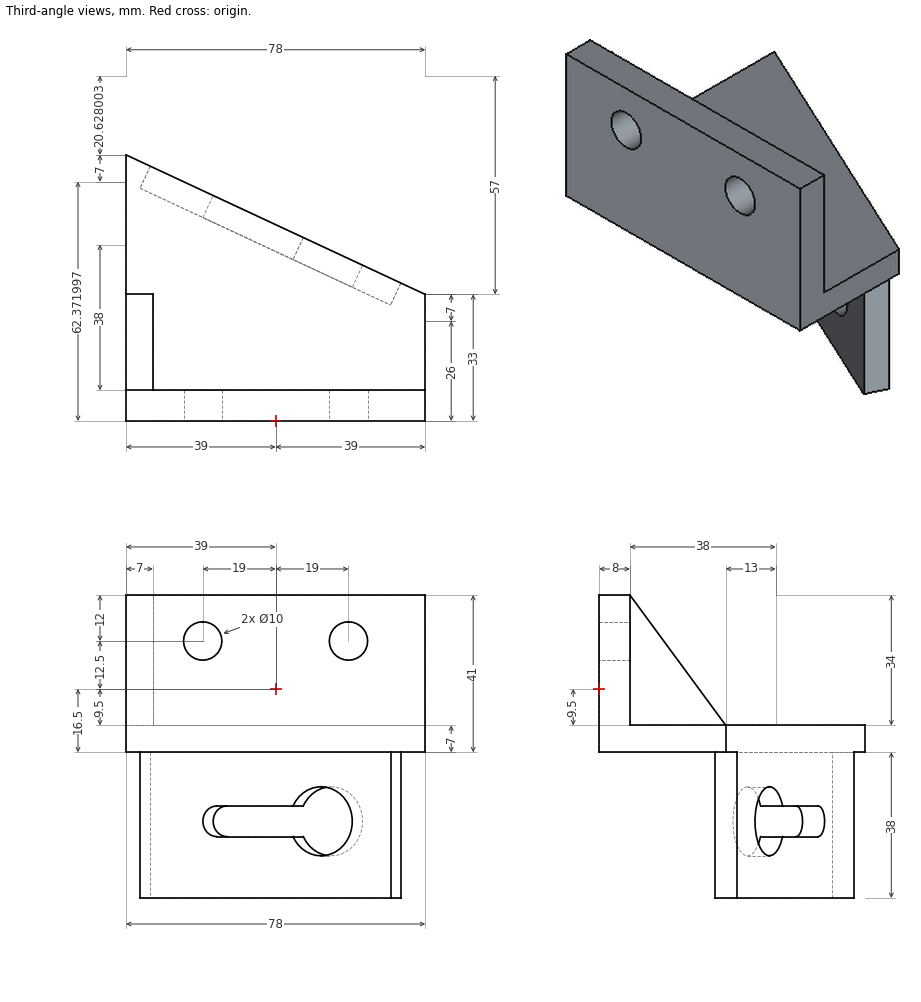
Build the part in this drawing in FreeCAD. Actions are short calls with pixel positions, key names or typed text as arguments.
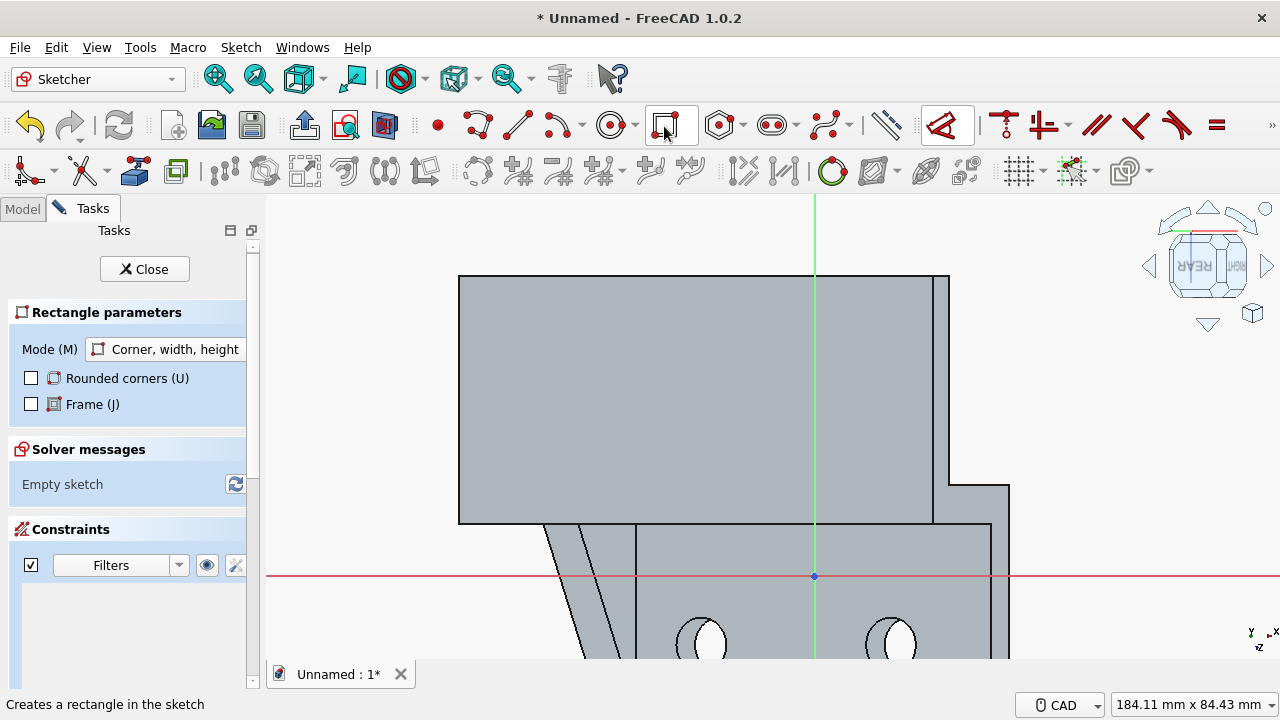
click(894, 276)
move(949, 485)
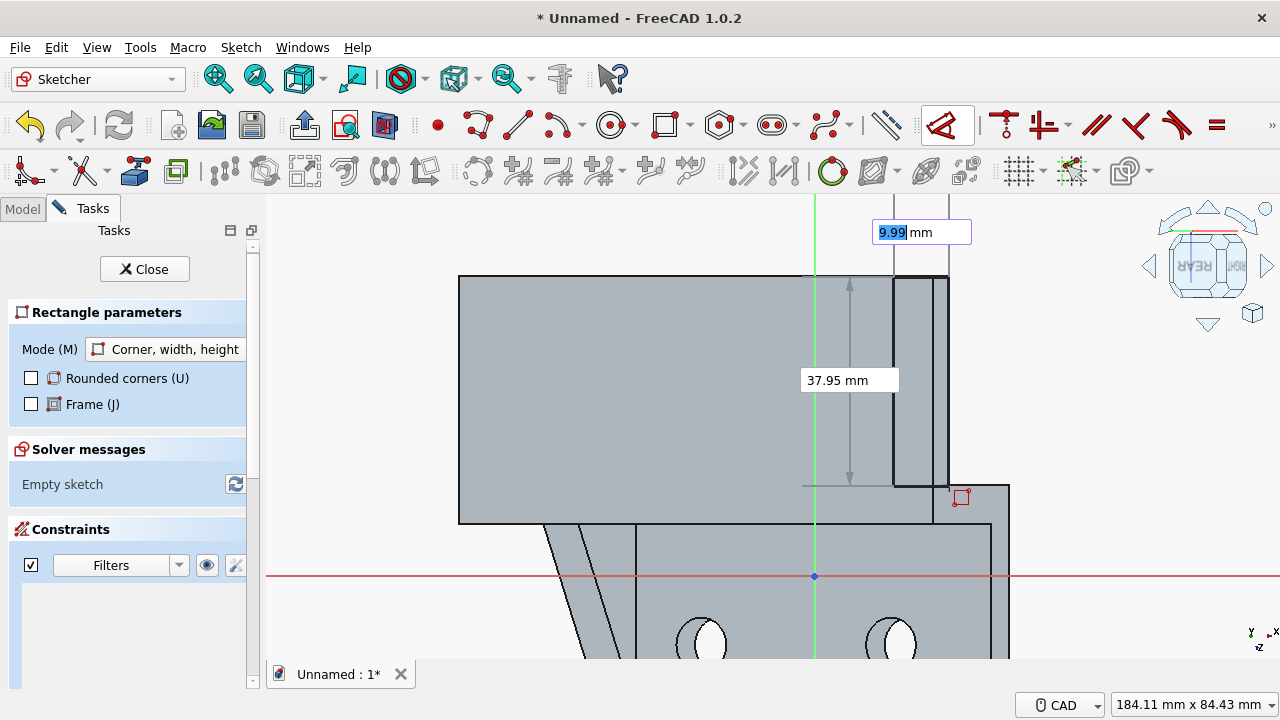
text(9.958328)
key(Tab)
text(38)
key(Return)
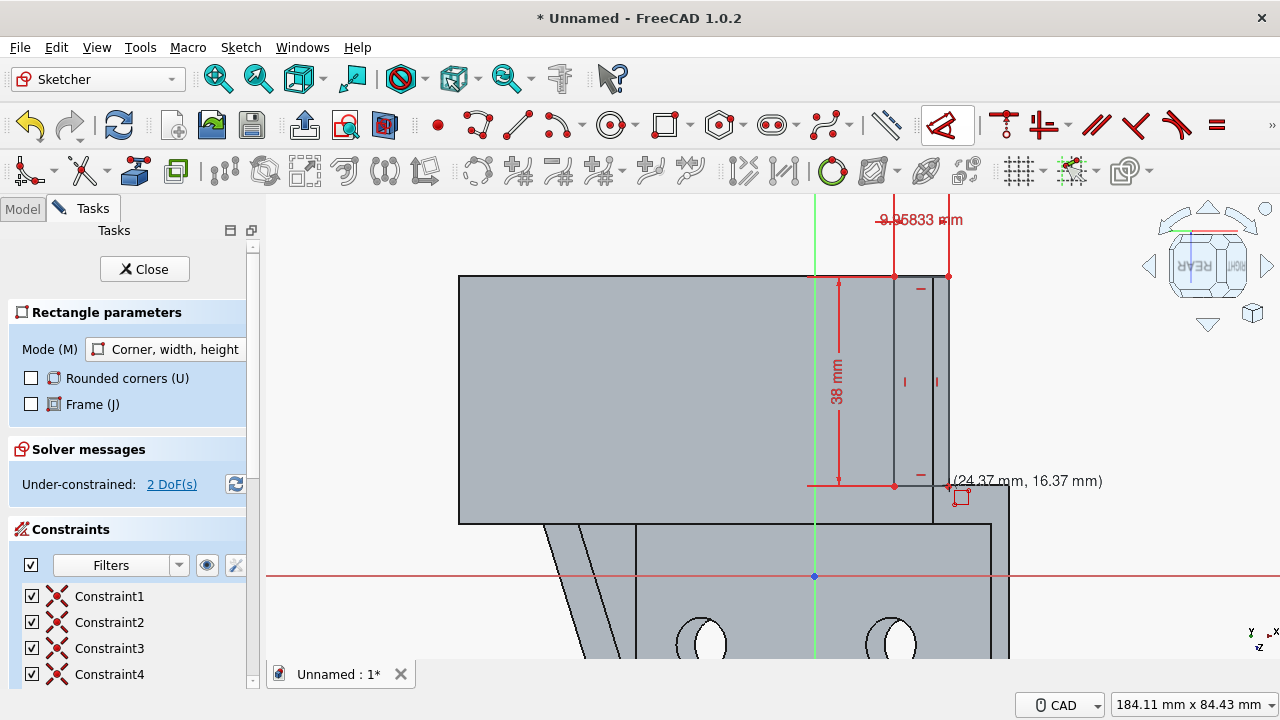
click(459, 276)
move(497, 485)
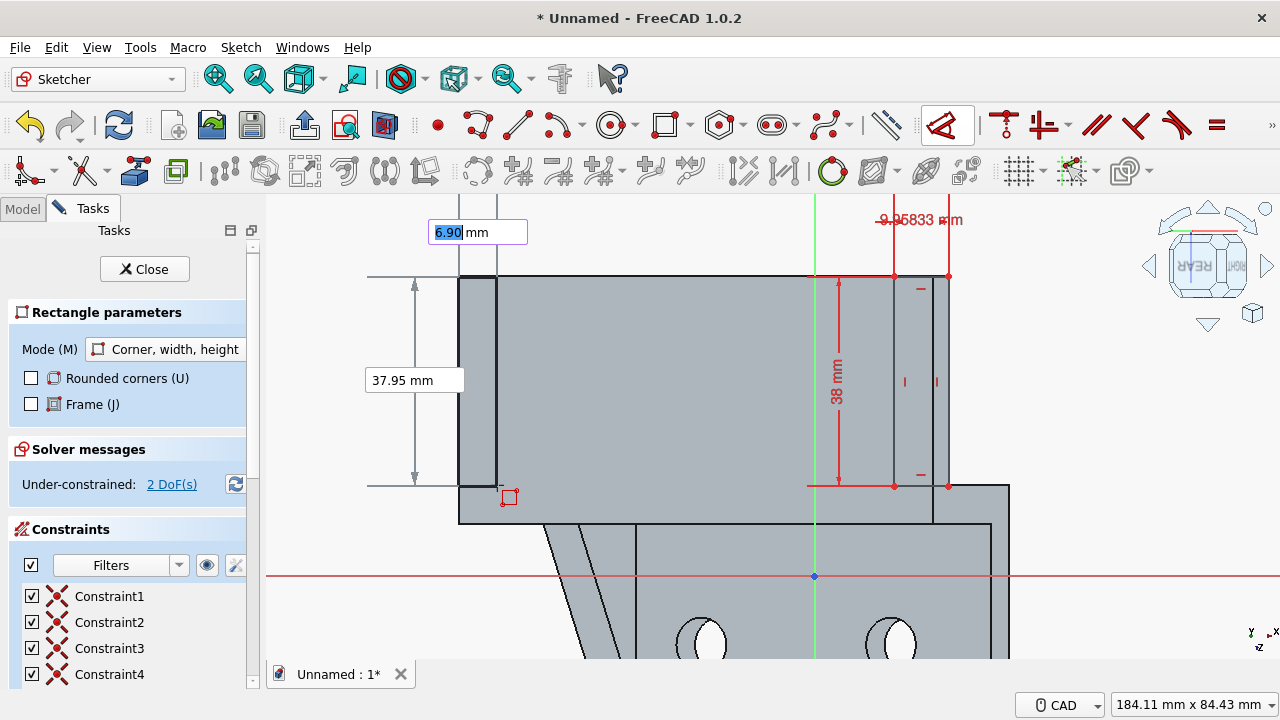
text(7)
key(Tab)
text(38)
key(Return)
key(Escape)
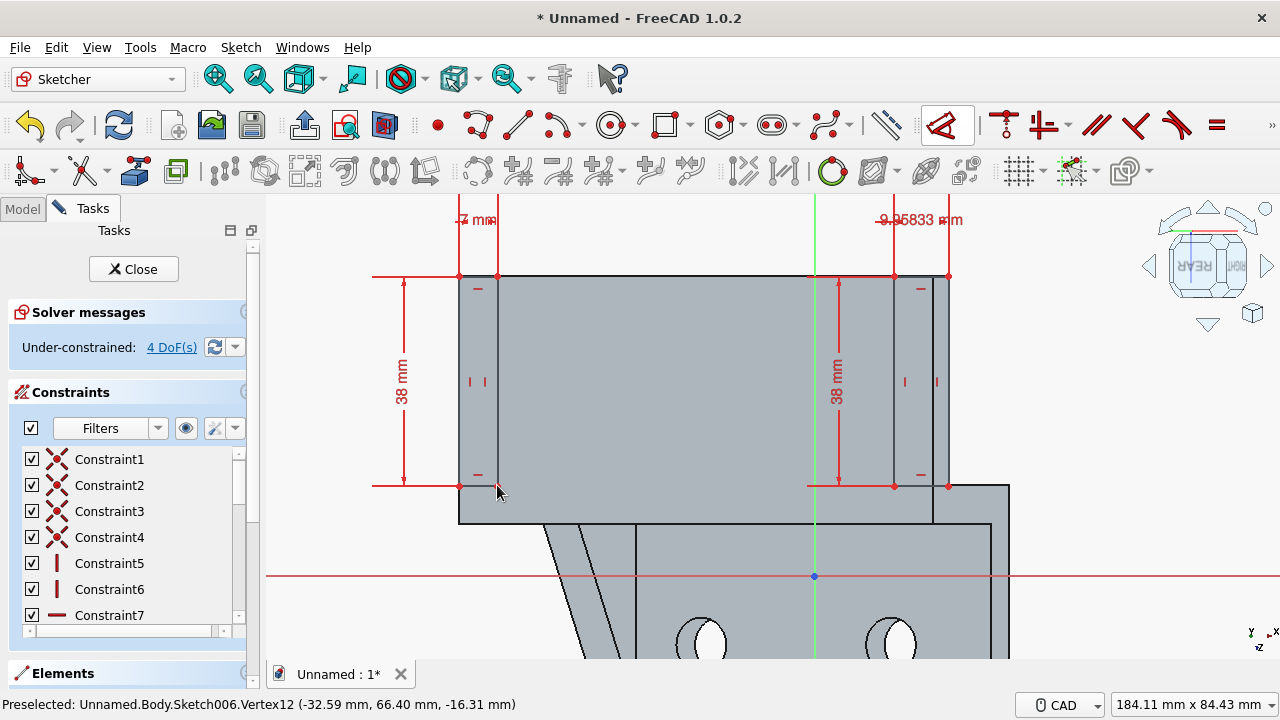
click(894, 277)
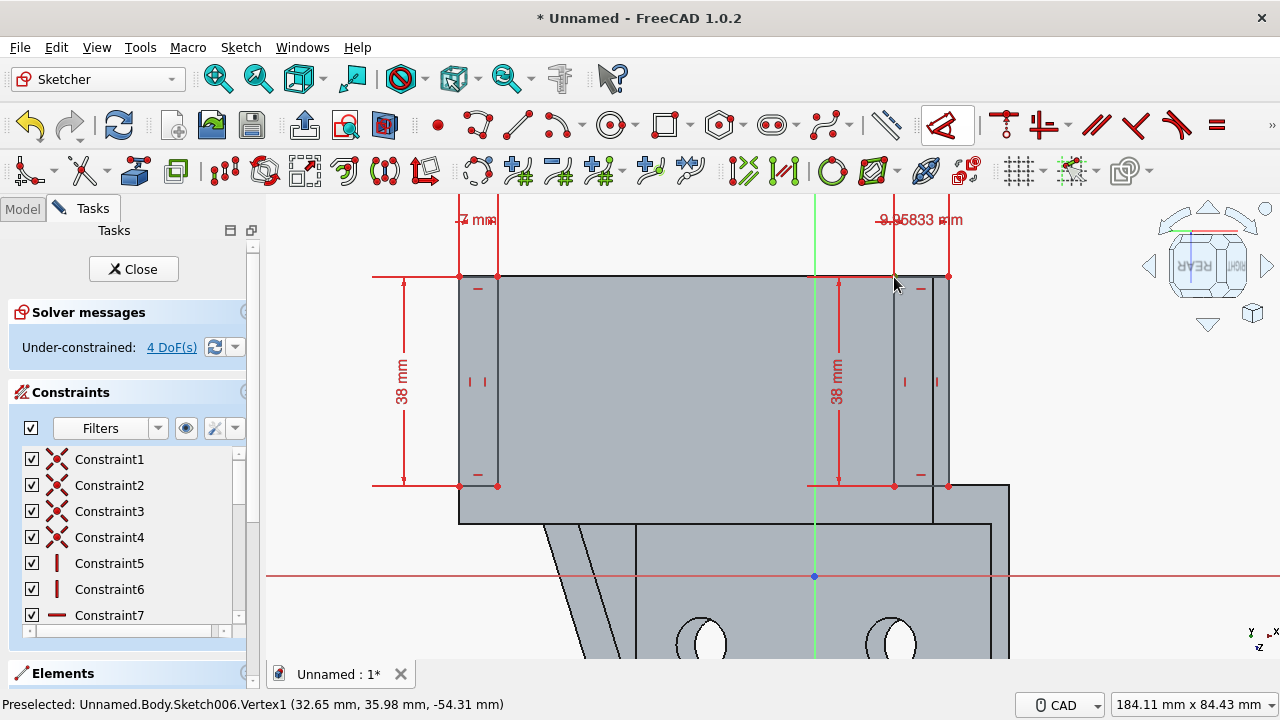
key(i)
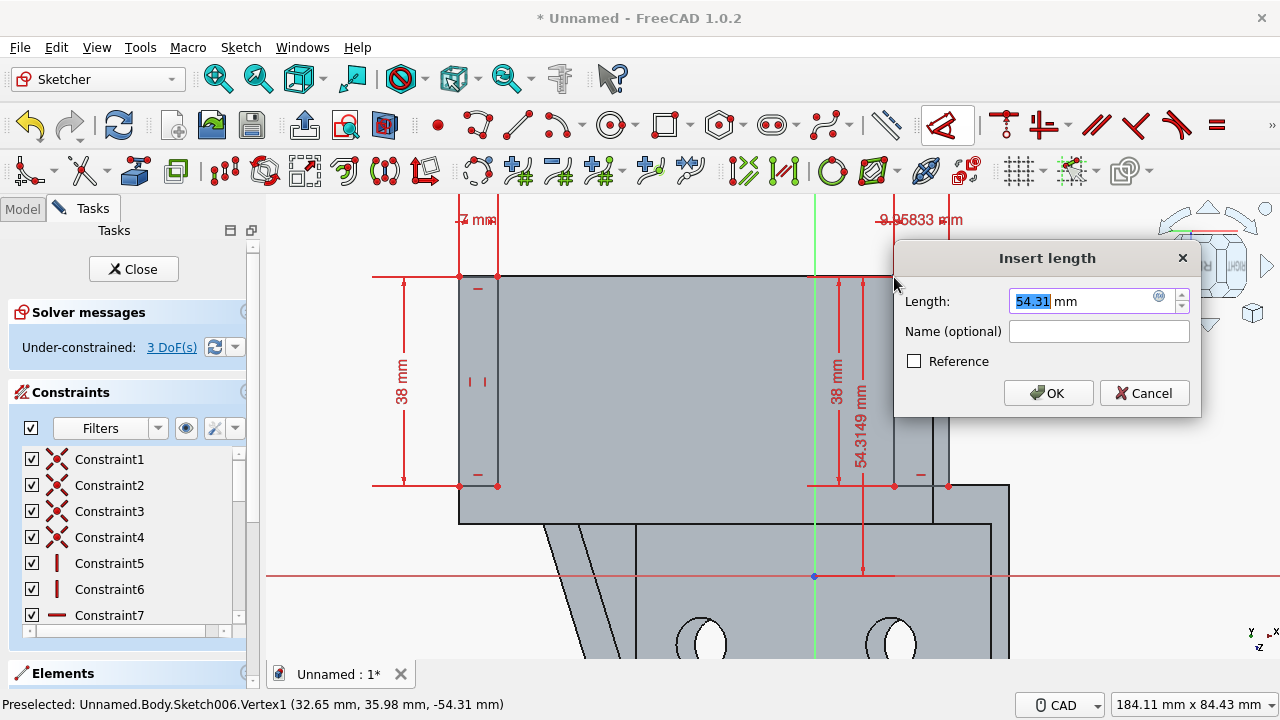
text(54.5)
key(Return)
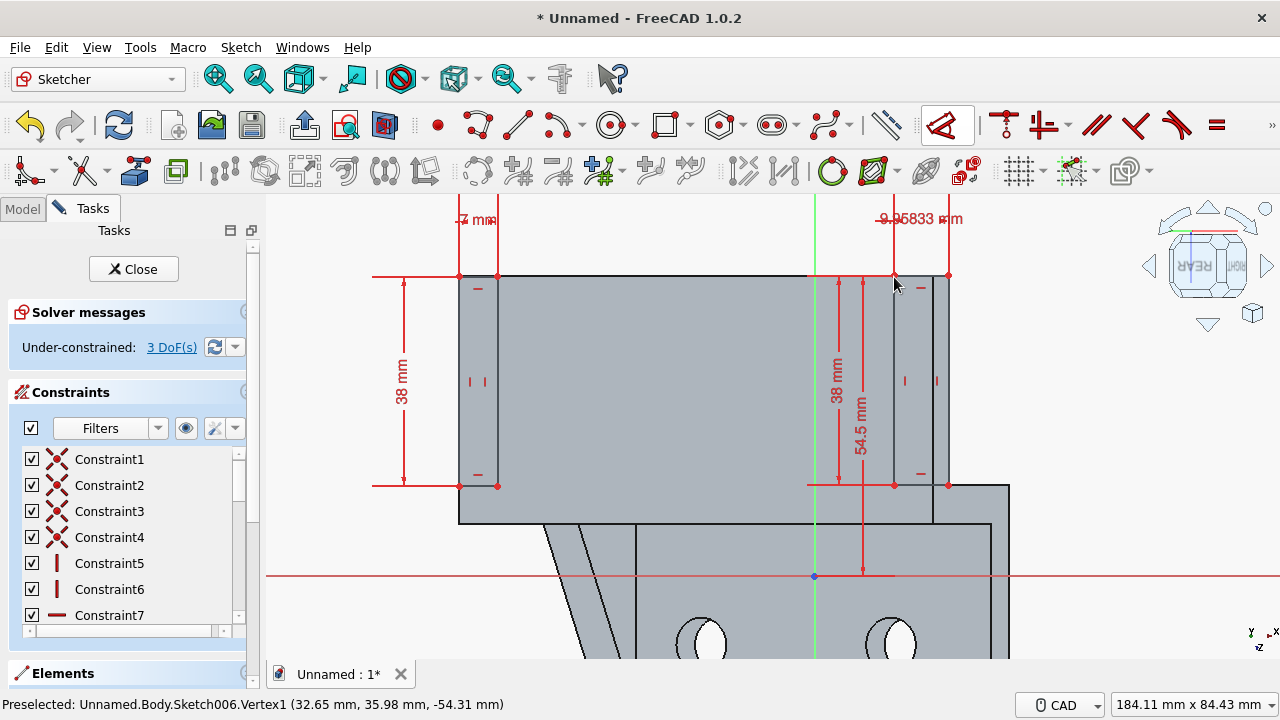
click(459, 277)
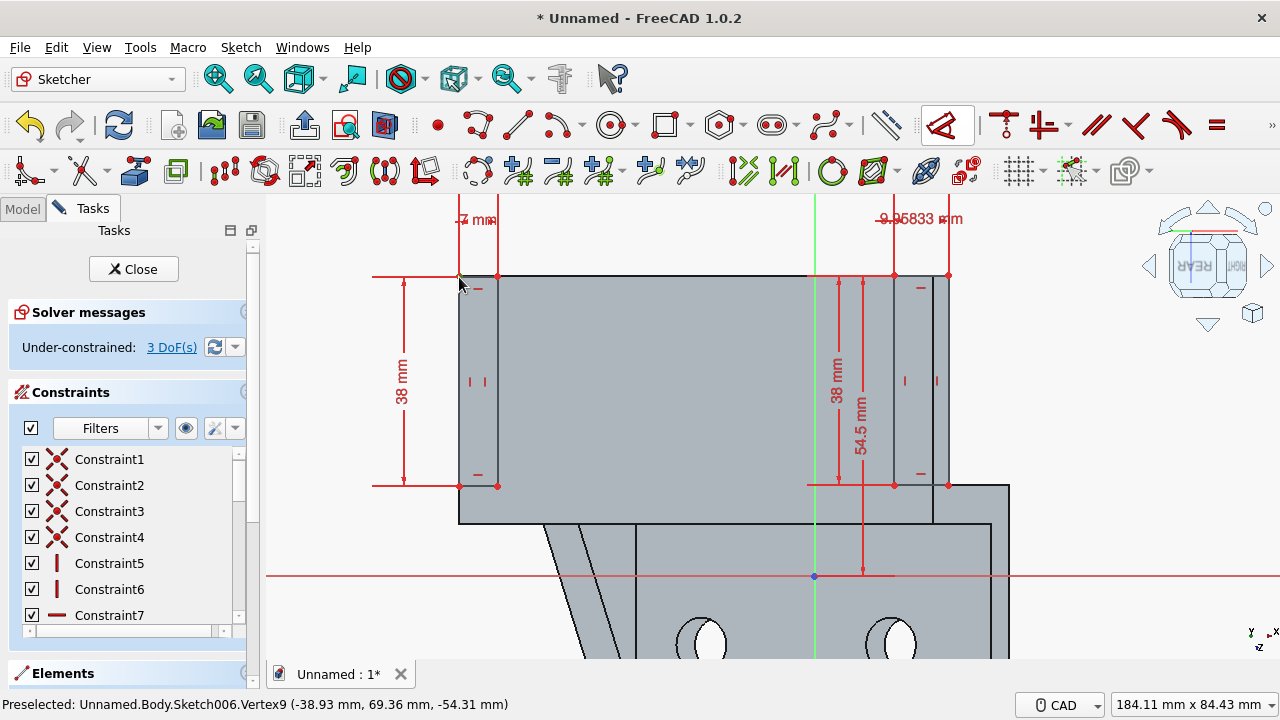
key(i)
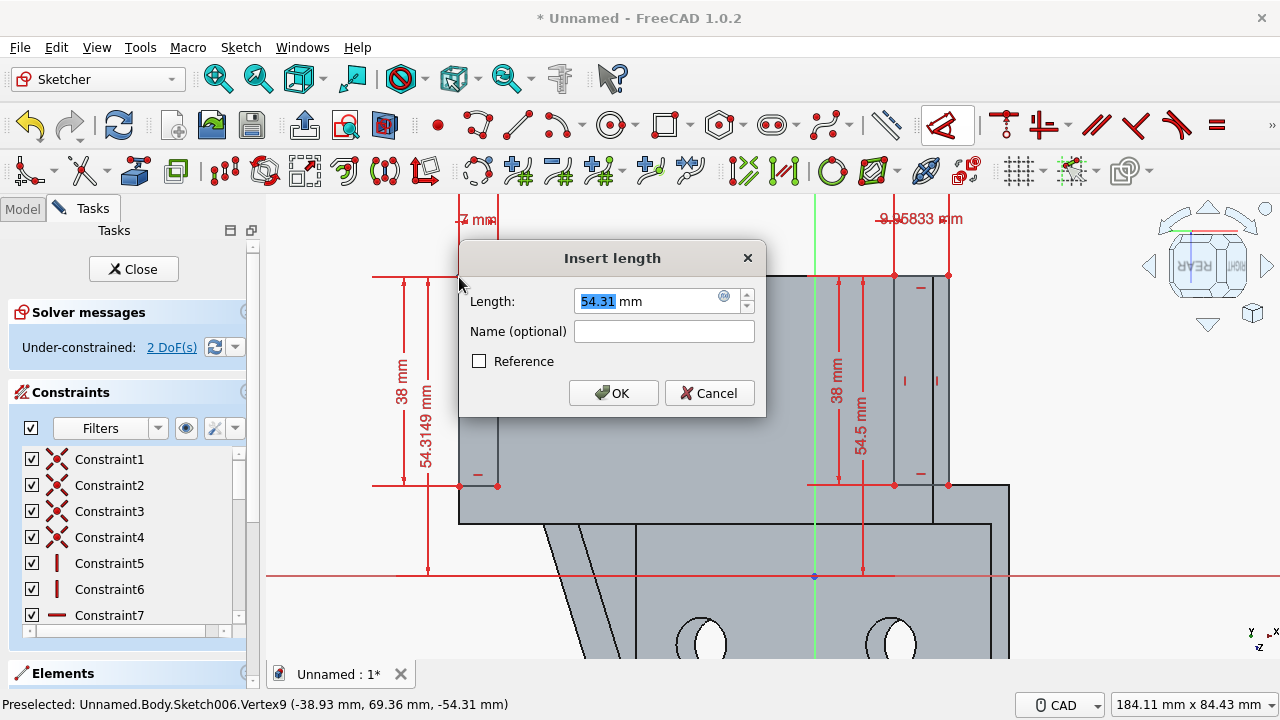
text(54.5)
key(Return)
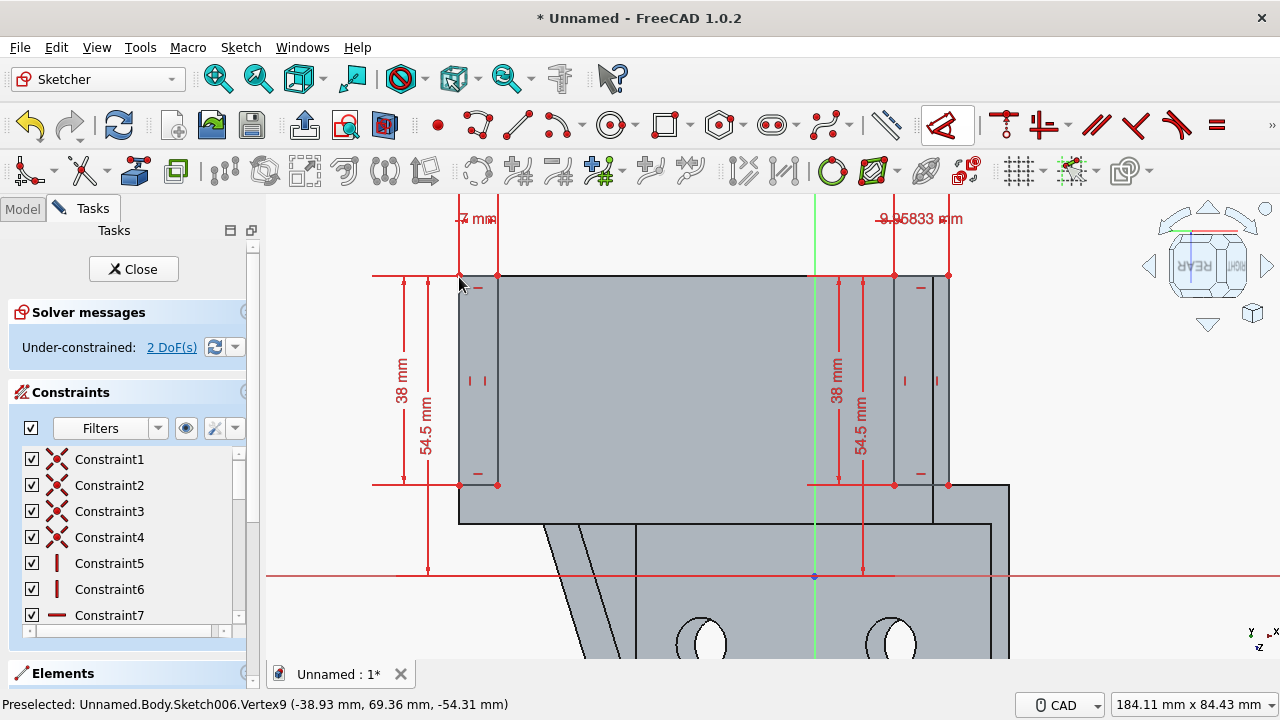
click(894, 276)